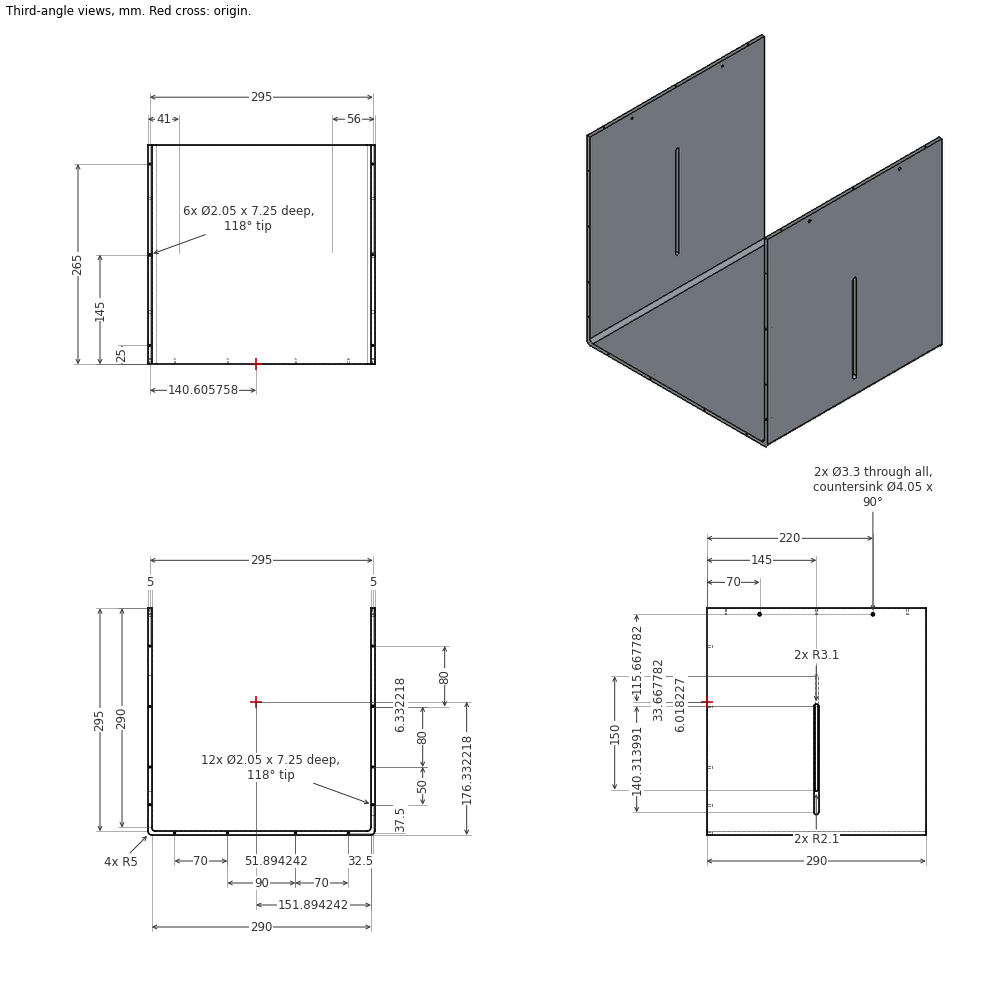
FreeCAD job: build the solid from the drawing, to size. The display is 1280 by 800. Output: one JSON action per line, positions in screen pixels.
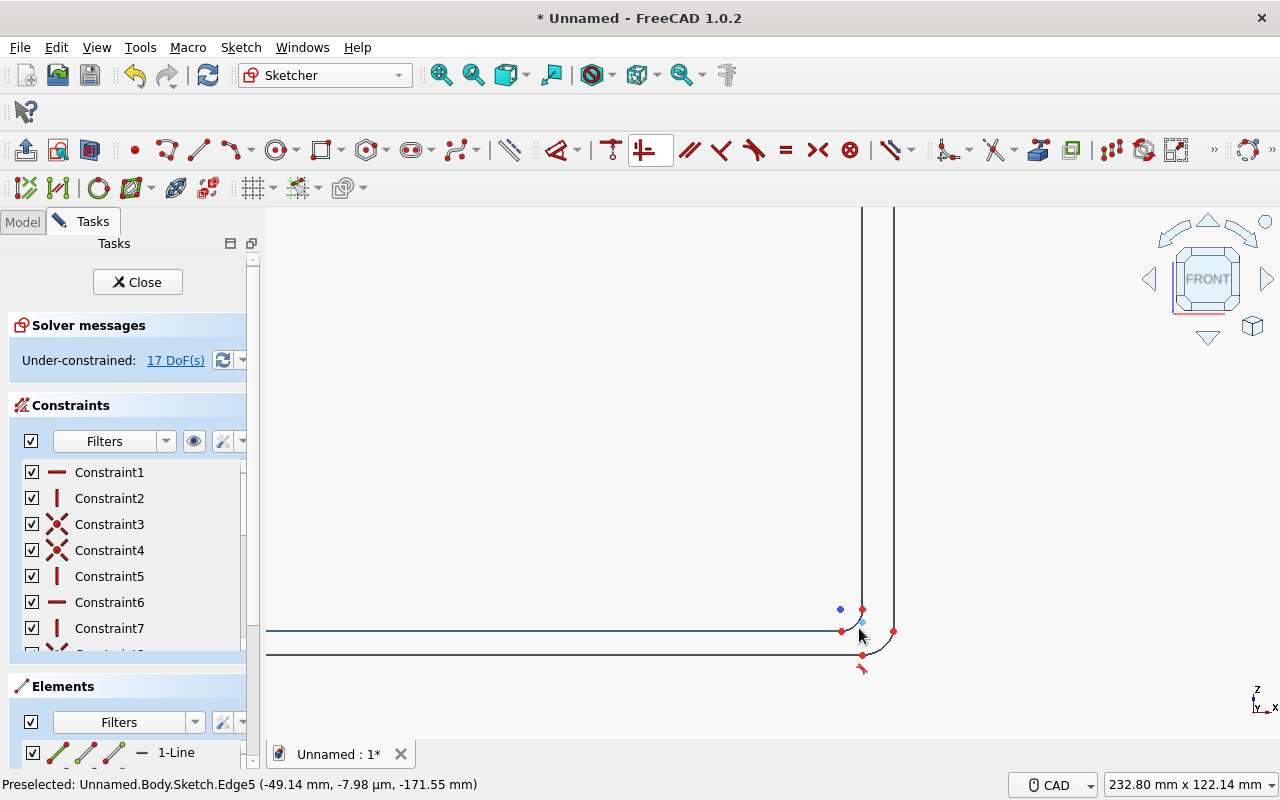
{"action": "left_click", "coordinate": [856, 625]}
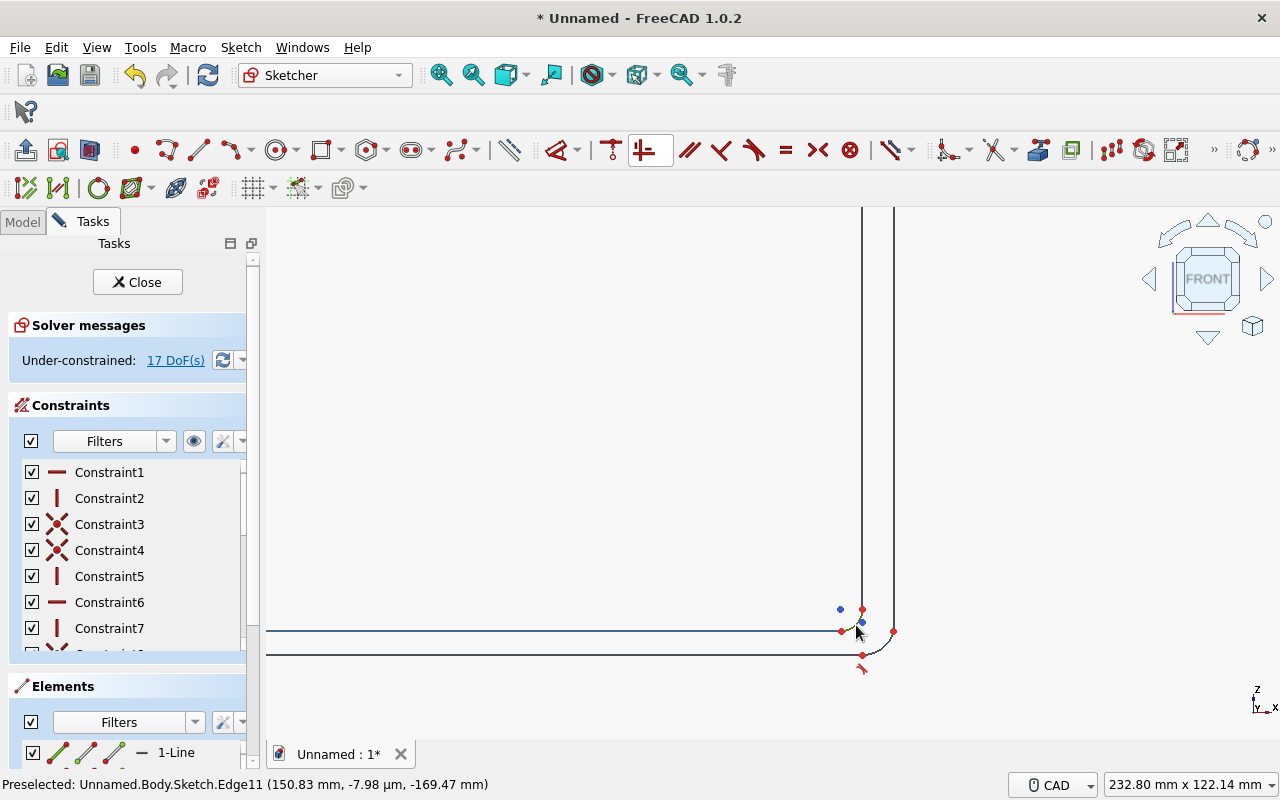
{"action": "left_click", "coordinate": [754, 150]}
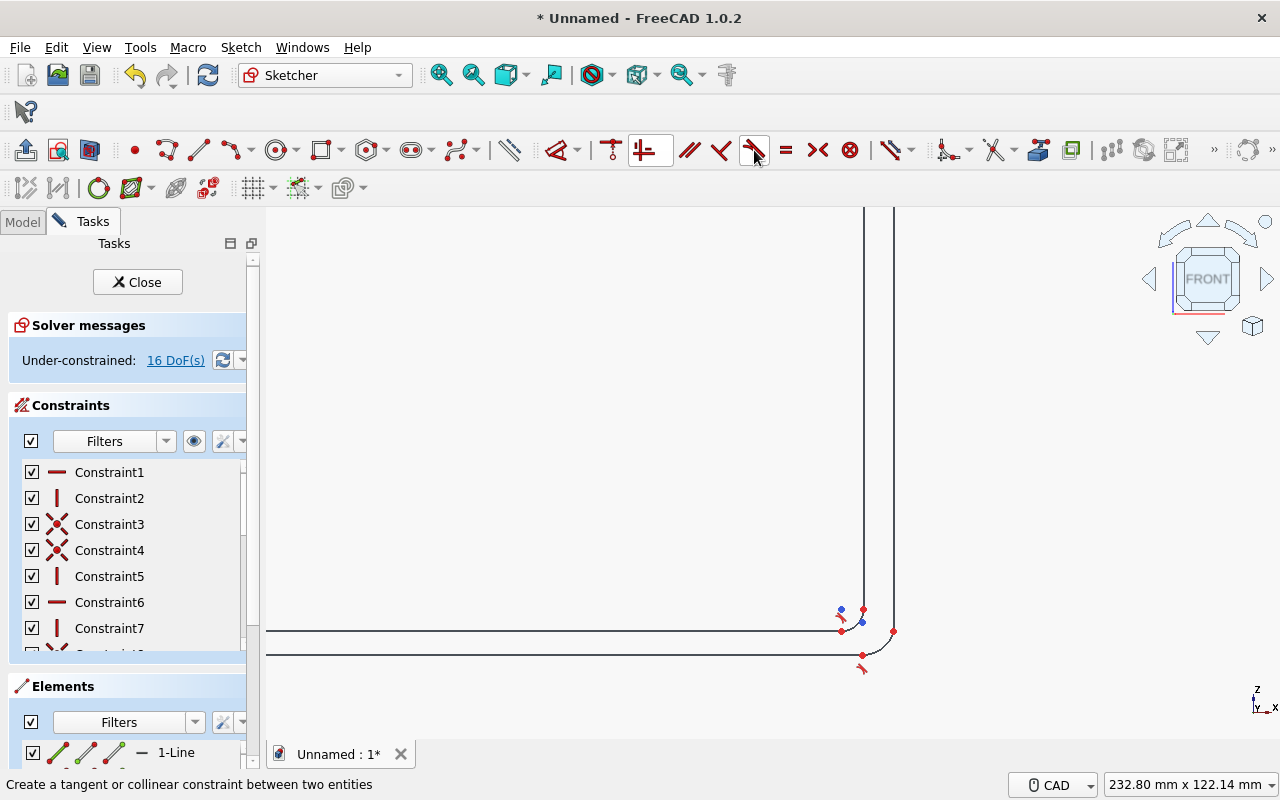
{"action": "left_click", "coordinate": [864, 358]}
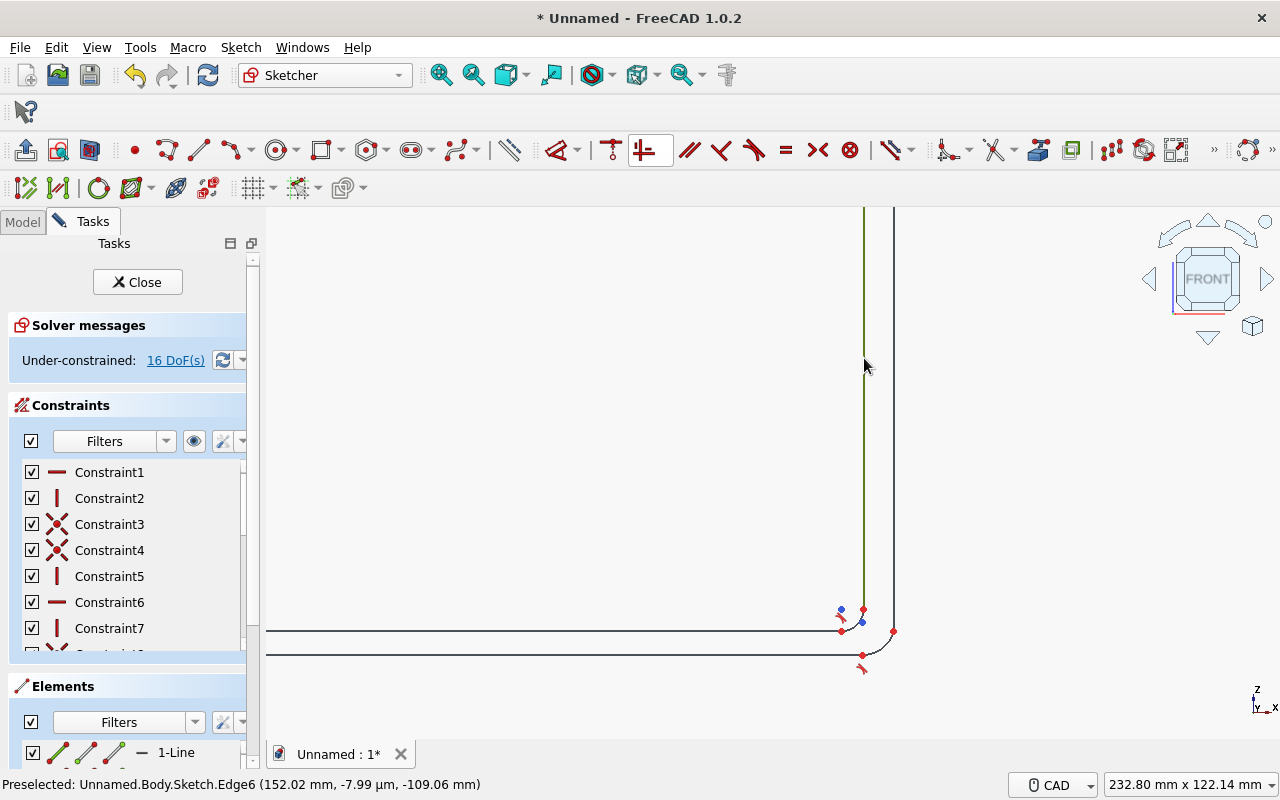
{"action": "scroll", "coordinate": [851, 629], "scroll_direction": "up", "scroll_amount": 2}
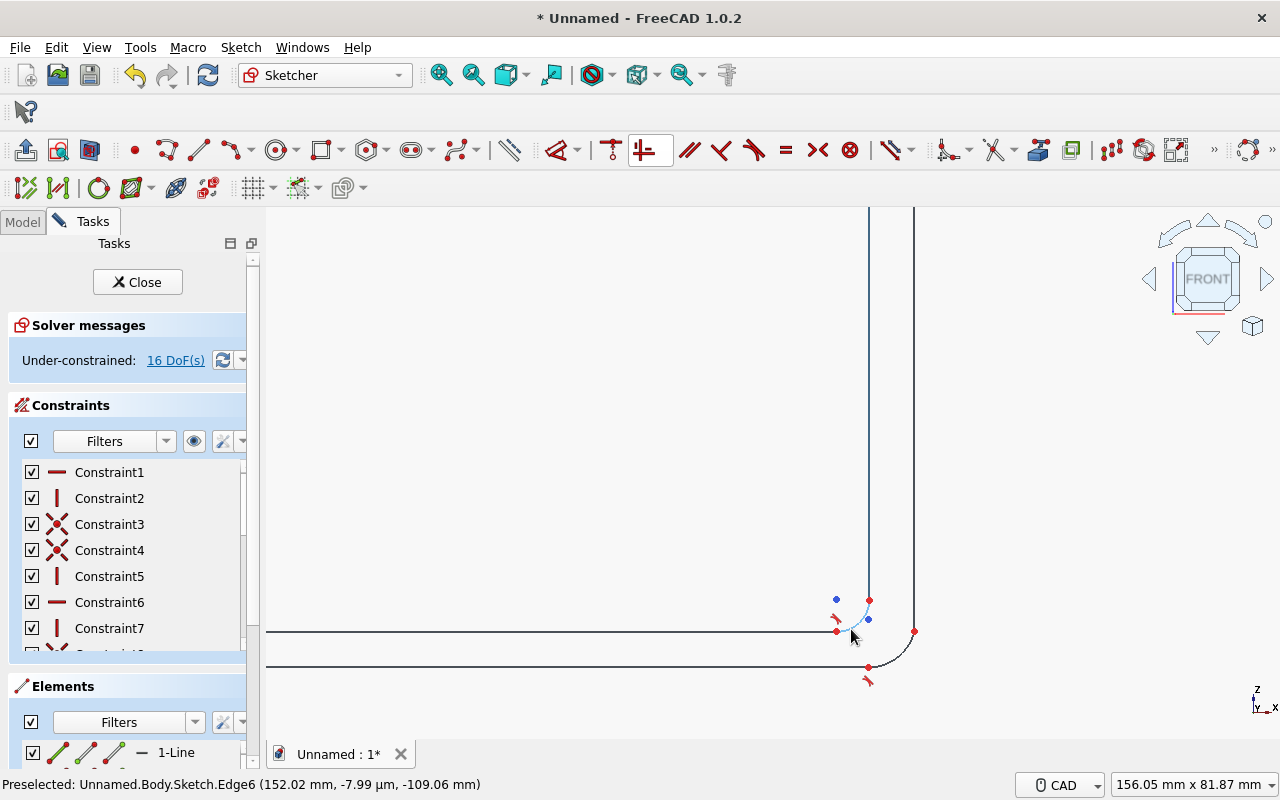
{"action": "left_click", "coordinate": [851, 628]}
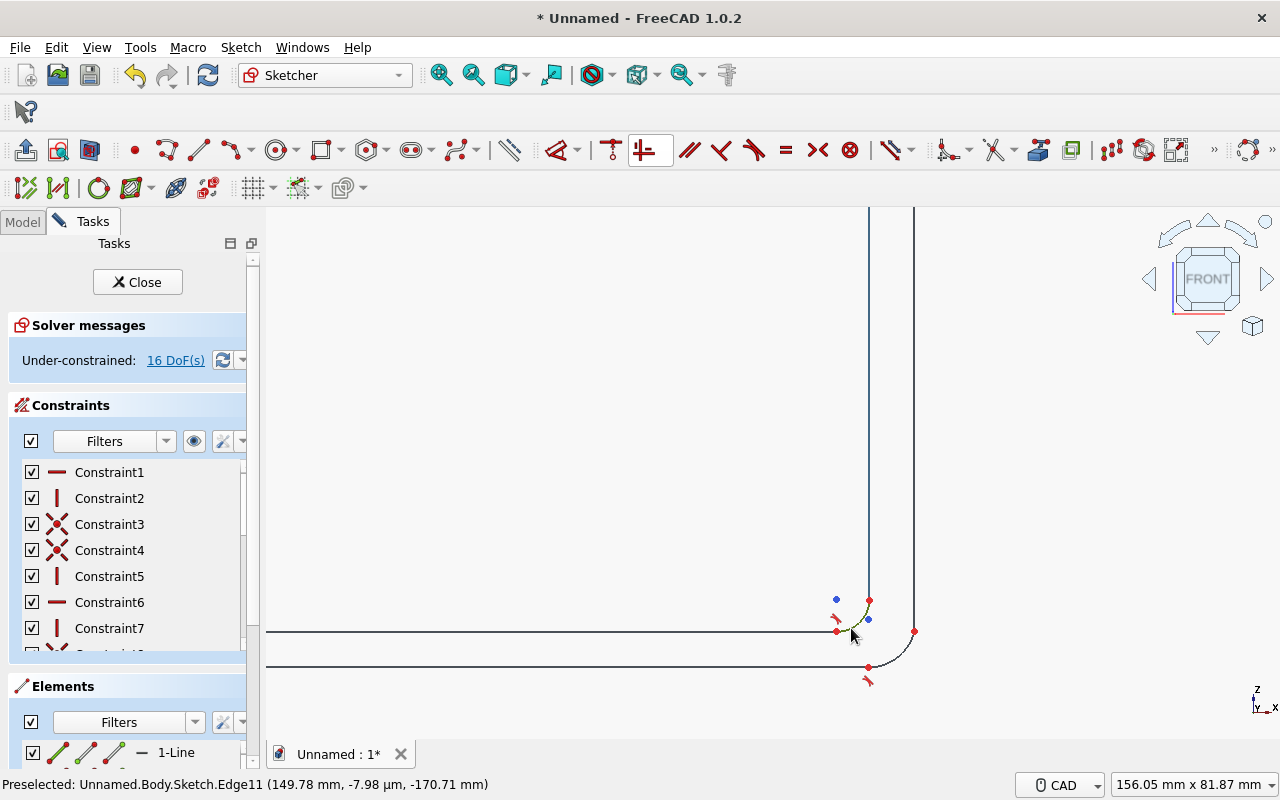
{"action": "left_click", "coordinate": [754, 150]}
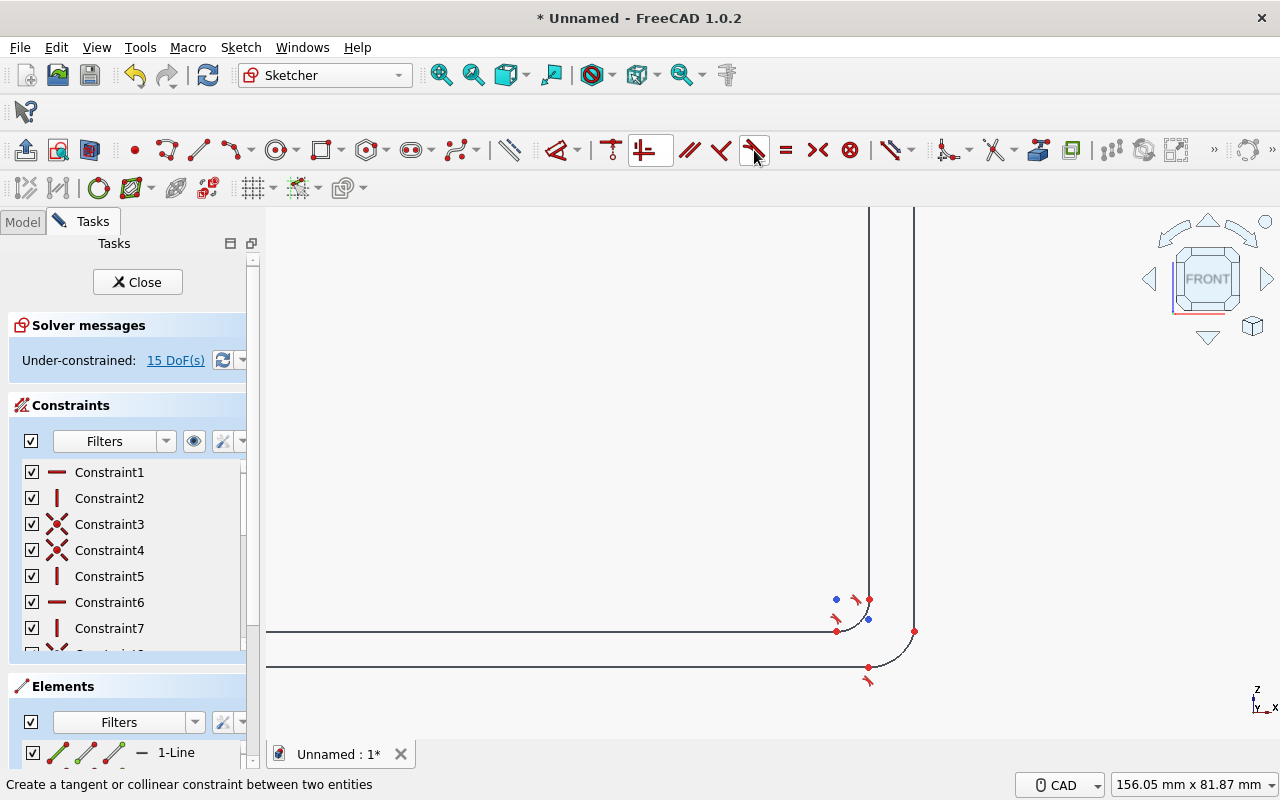
{"action": "scroll", "coordinate": [859, 628], "scroll_direction": "down", "scroll_amount": 9}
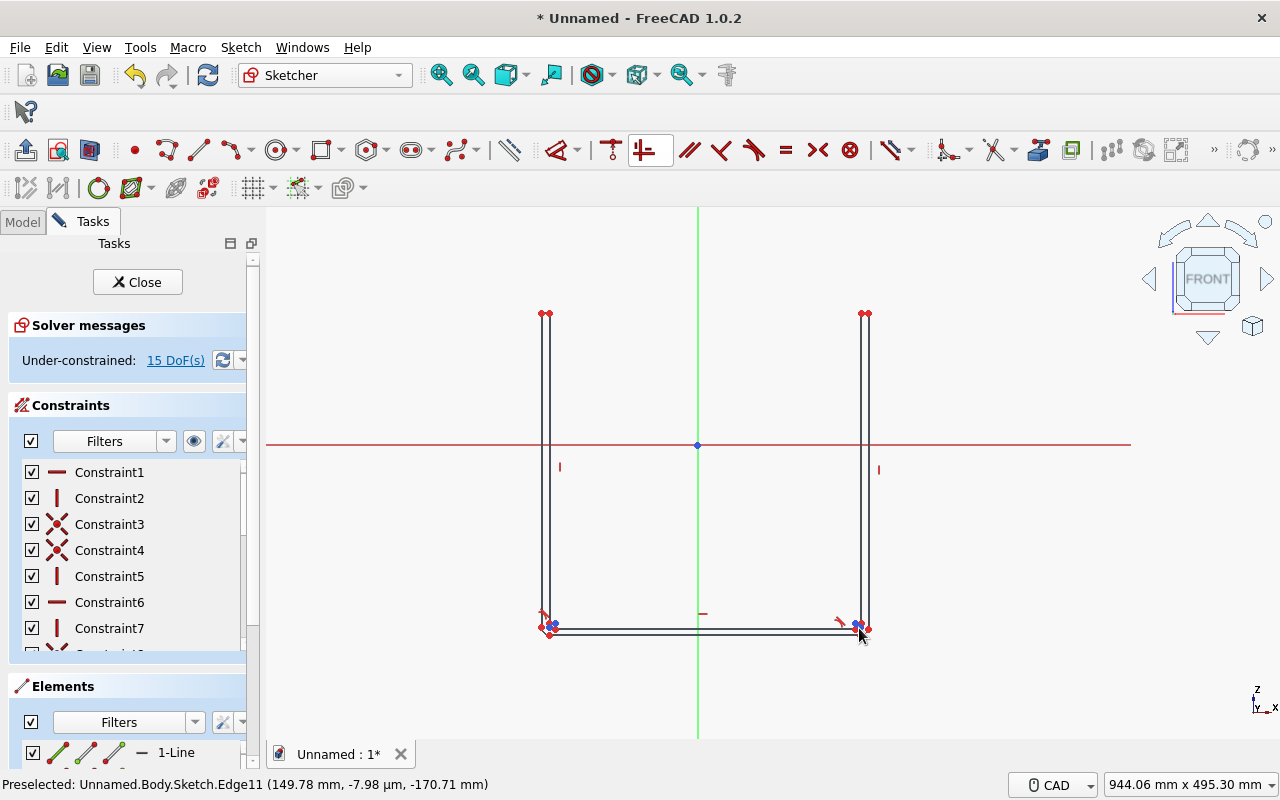
{"action": "scroll", "coordinate": [869, 566], "scroll_direction": "up", "scroll_amount": 4}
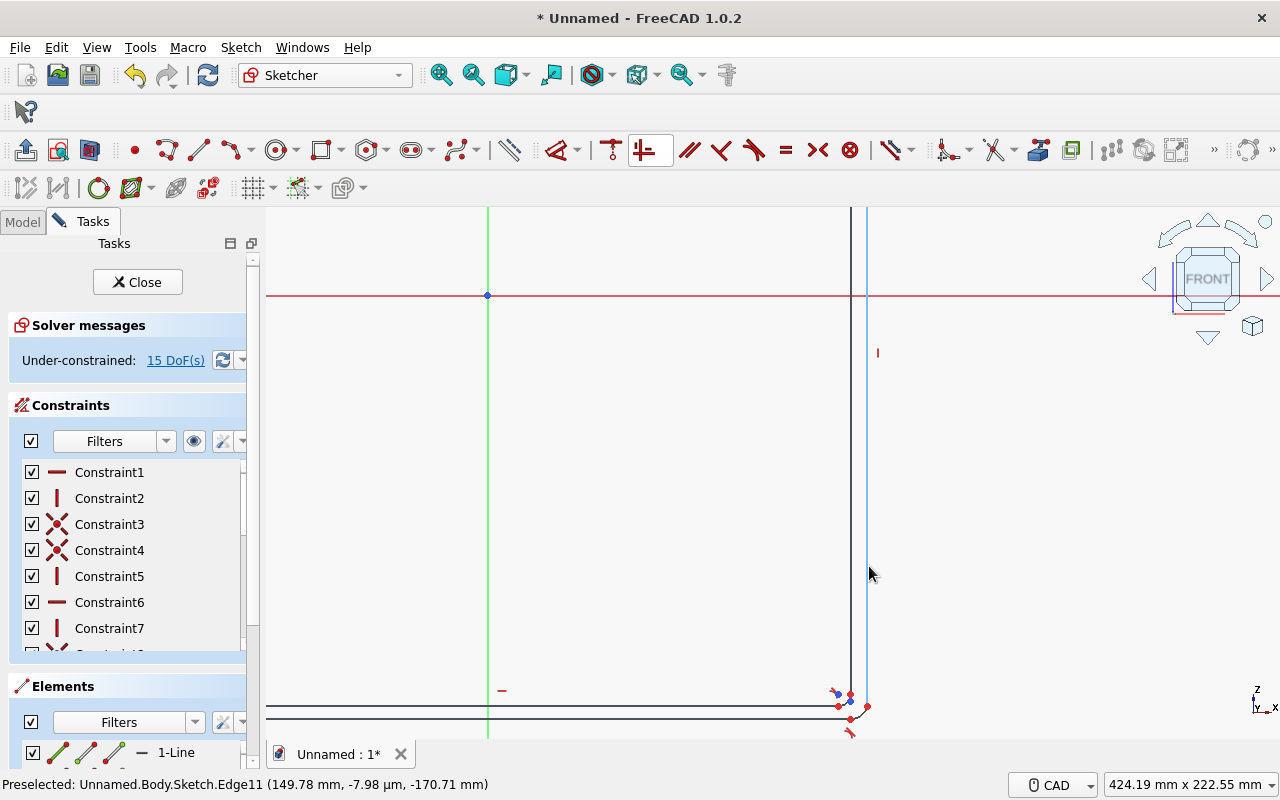
{"action": "left_click", "coordinate": [867, 565]}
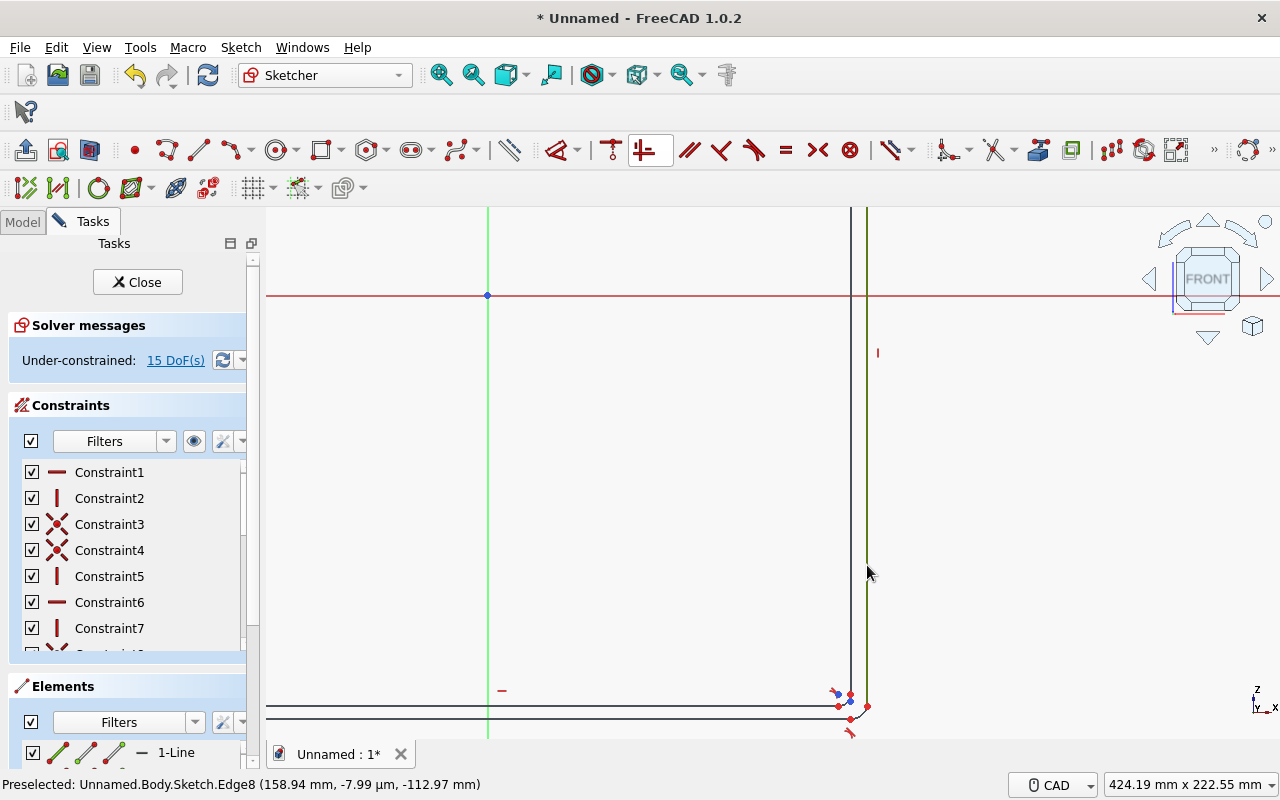
{"action": "scroll", "coordinate": [868, 566], "scroll_direction": "down", "scroll_amount": 4}